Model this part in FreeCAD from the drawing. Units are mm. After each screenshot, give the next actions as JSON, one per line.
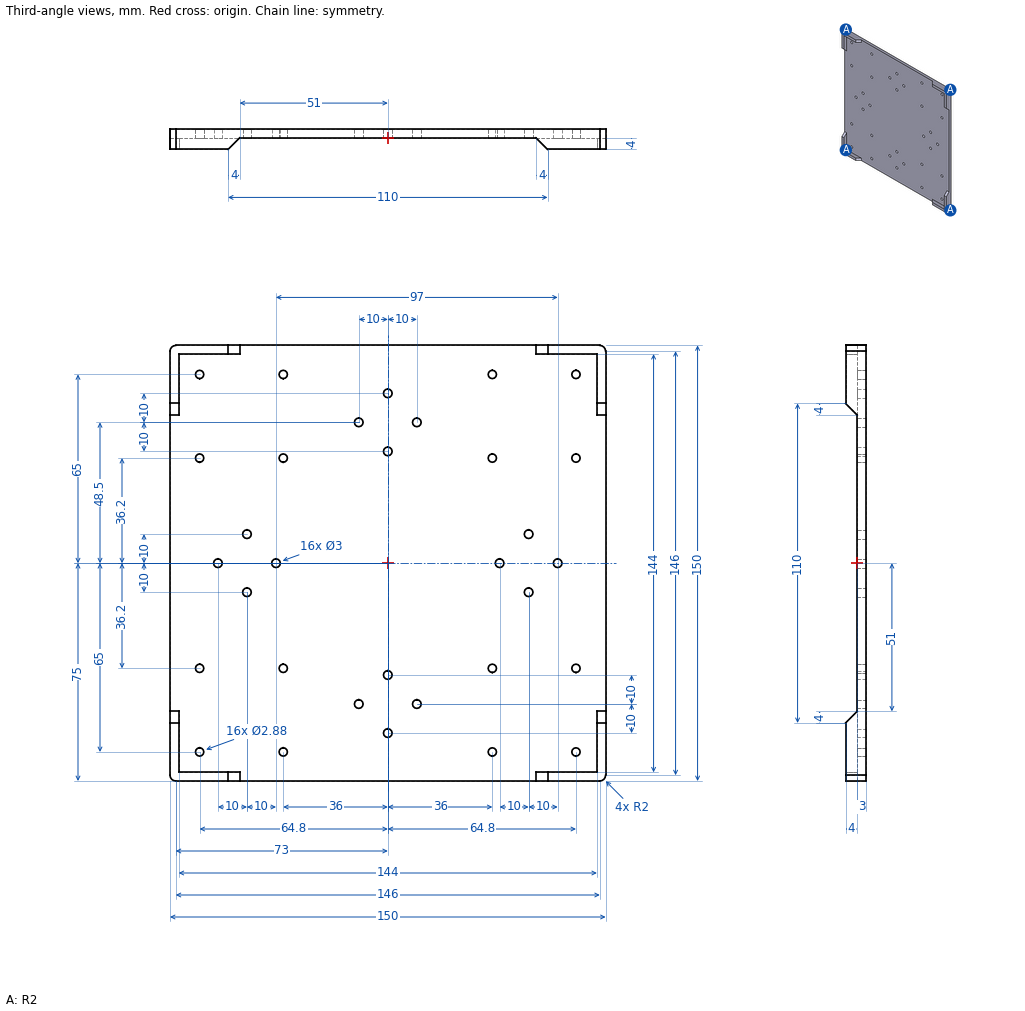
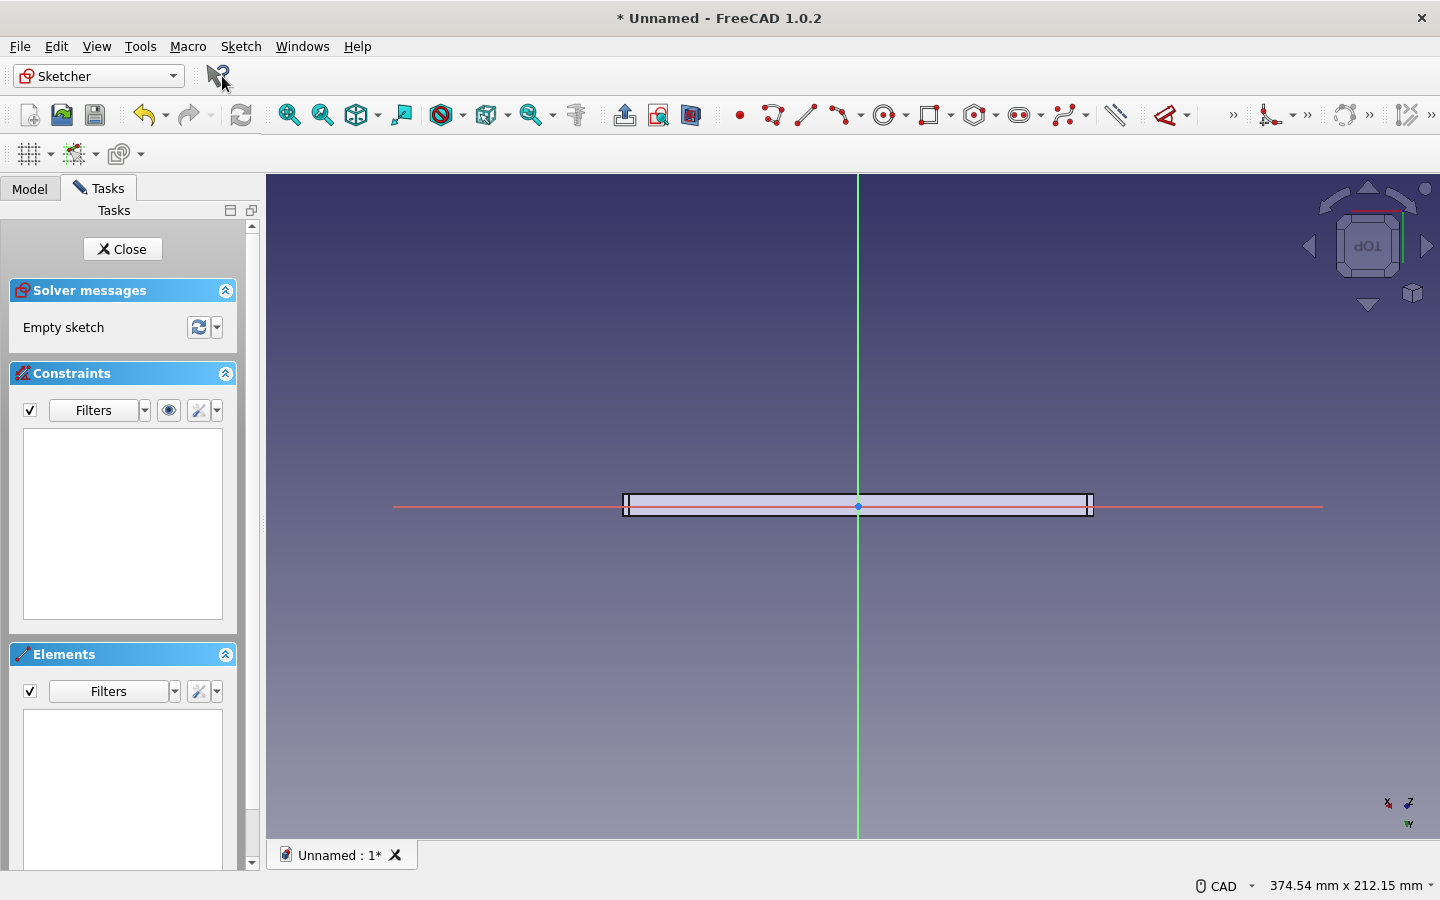
{"action": "scroll", "coordinate": [948, 493], "scroll_direction": "up", "scroll_amount": 3}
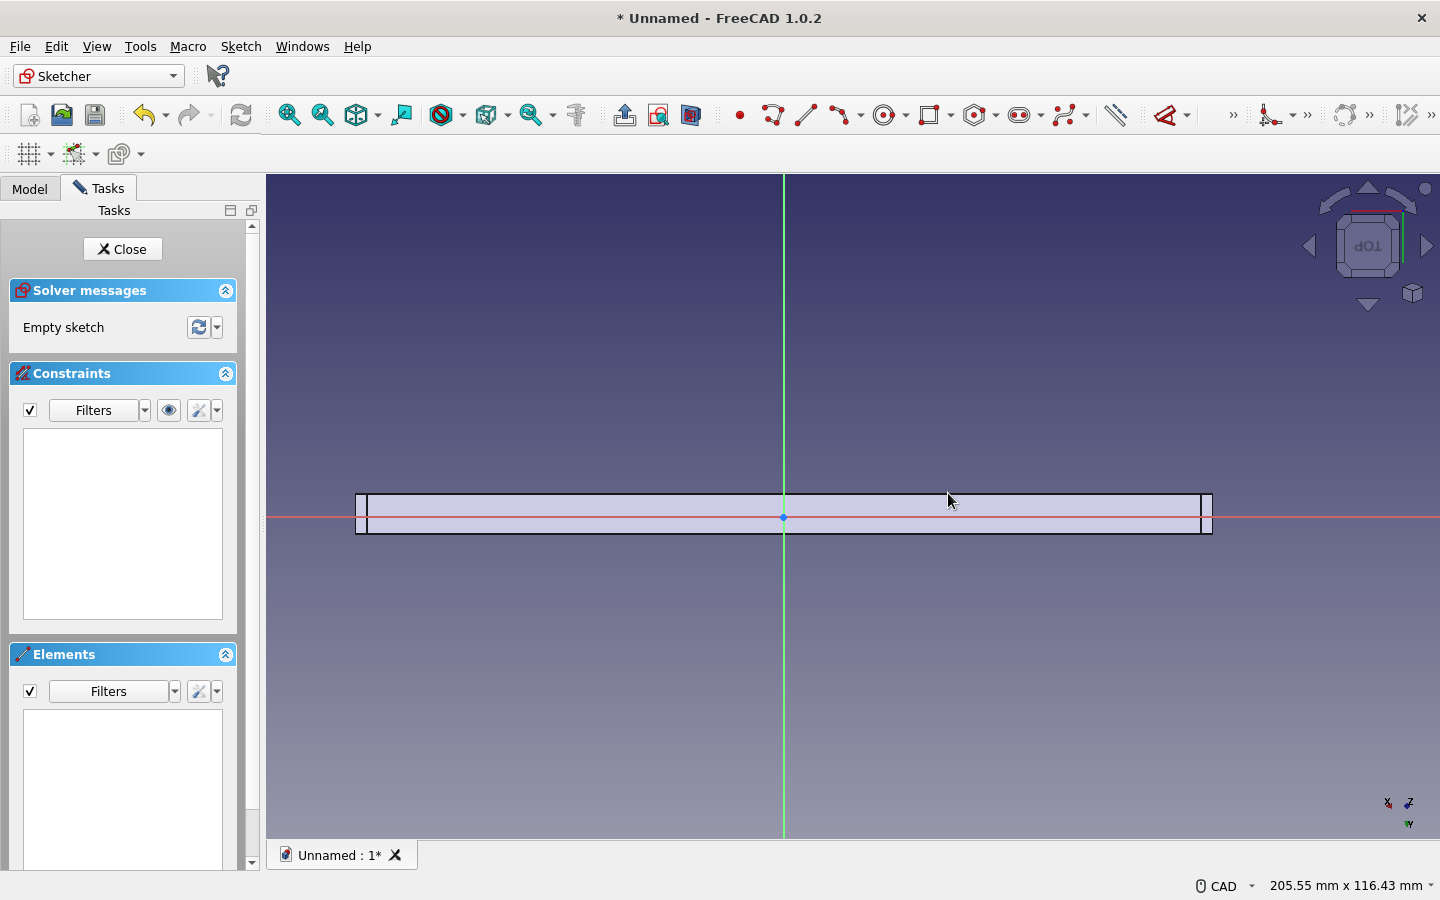
{"action": "key", "text": "g m"}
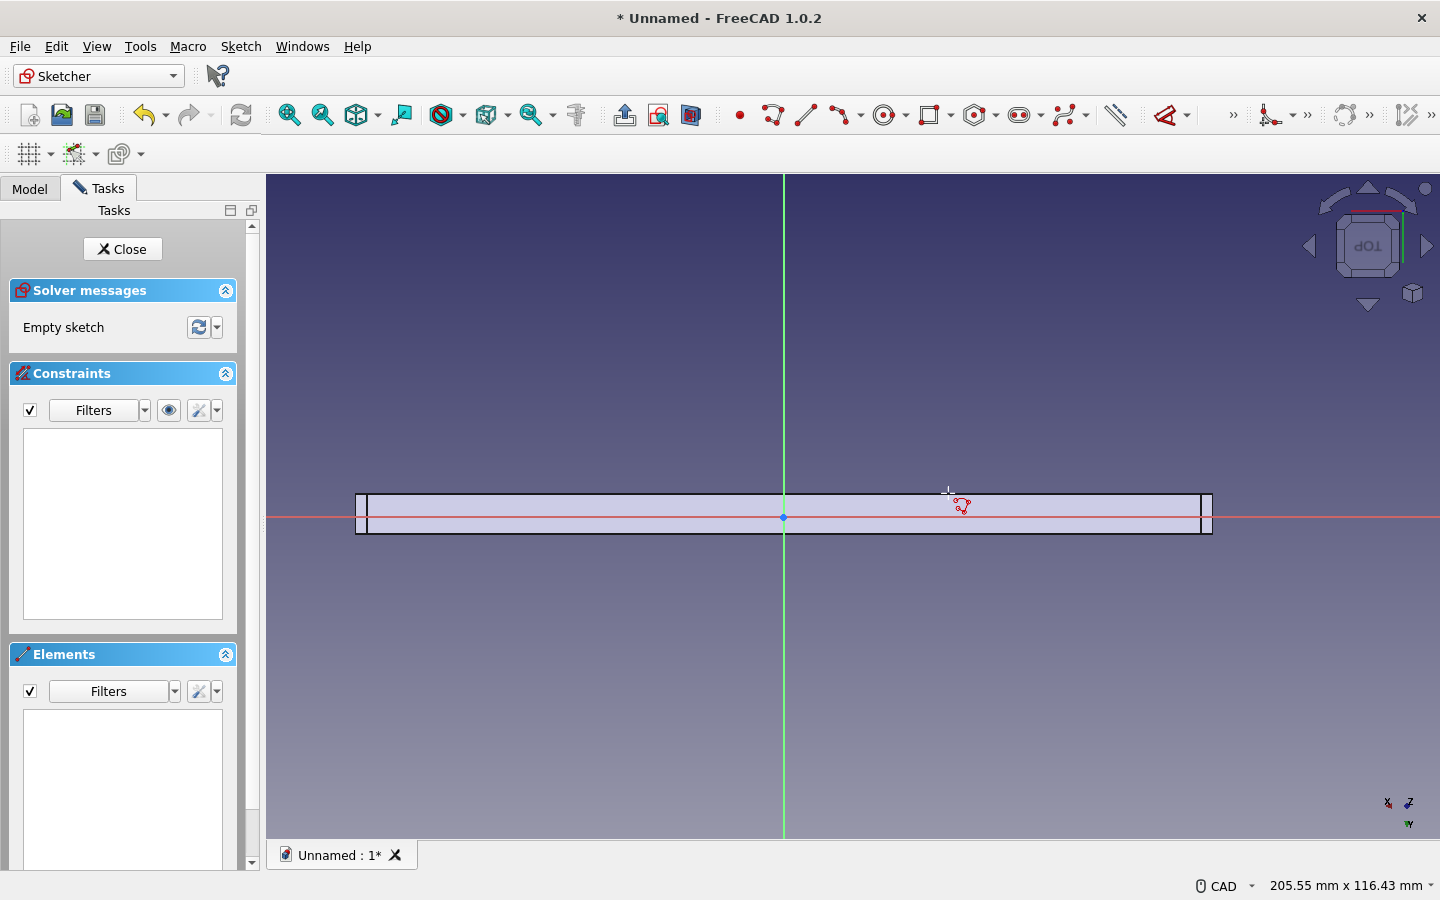
{"action": "left_click", "coordinate": [1075, 517]}
{"action": "left_click", "coordinate": [1098, 494]}
{"action": "left_click", "coordinate": [470, 494]}
{"action": "left_click", "coordinate": [493, 508]}
{"action": "left_click", "coordinate": [1075, 517]}
{"action": "key", "text": "Escape"}
{"action": "key", "text": "Escape"}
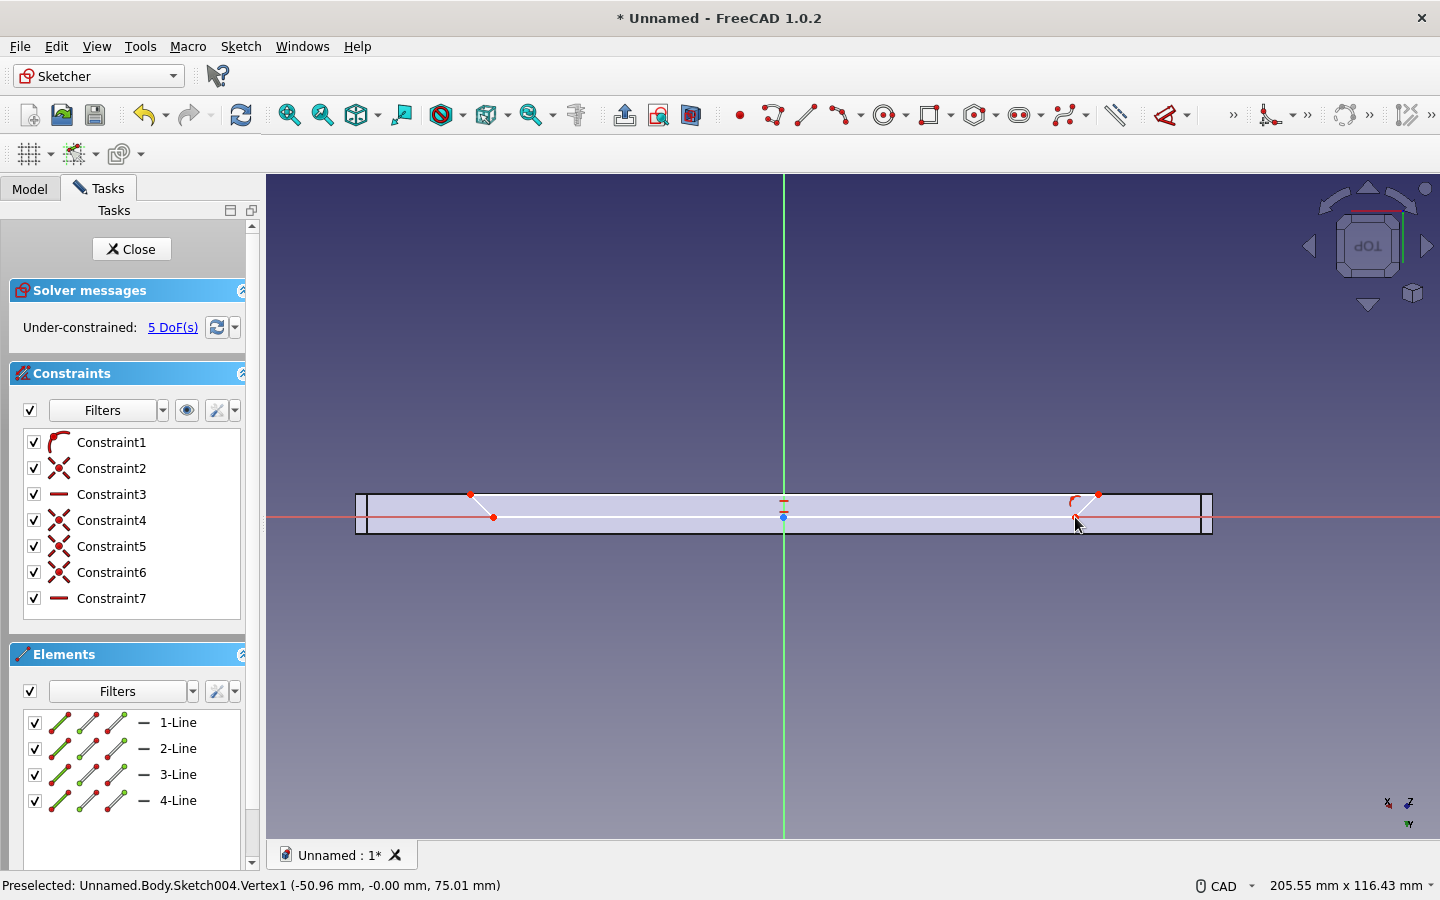
{"action": "left_click", "coordinate": [1164, 116]}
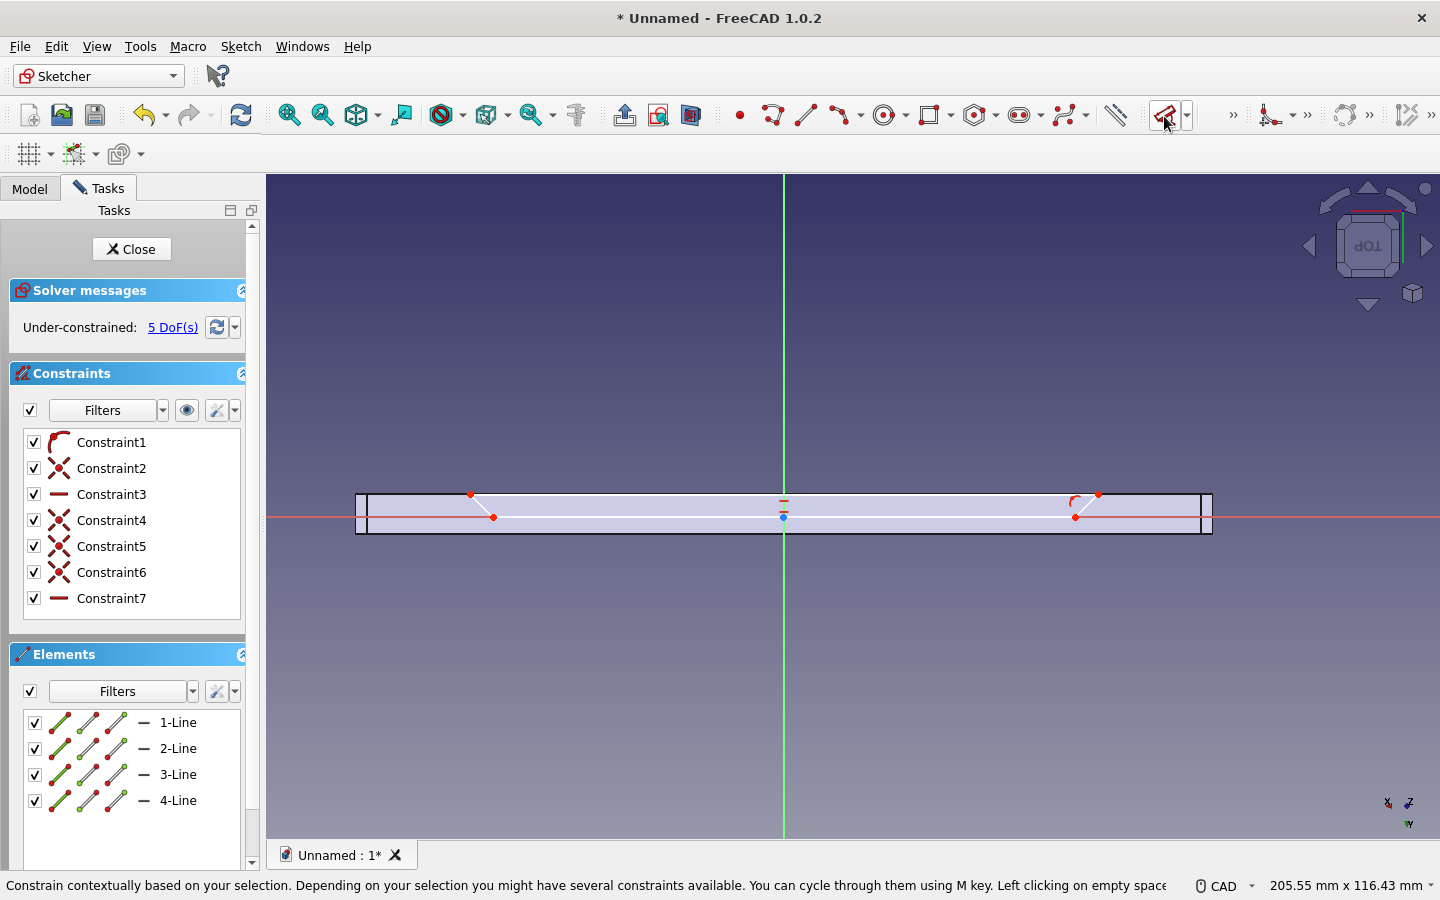
{"action": "scroll", "coordinate": [1098, 495], "scroll_direction": "up", "scroll_amount": 3}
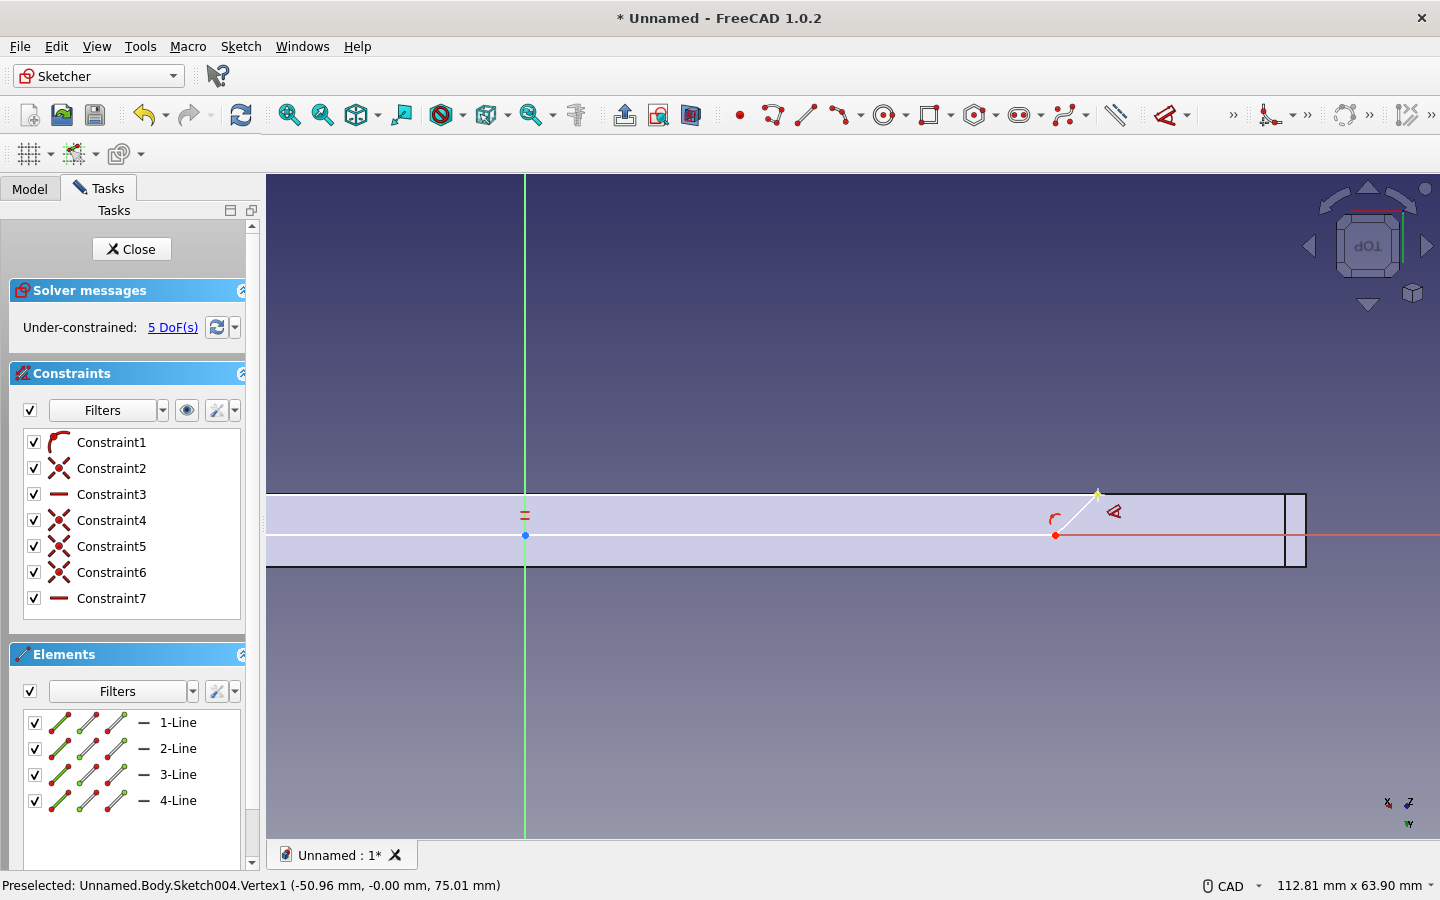
{"action": "left_click", "coordinate": [1097, 495]}
{"action": "left_click", "coordinate": [1131, 515]}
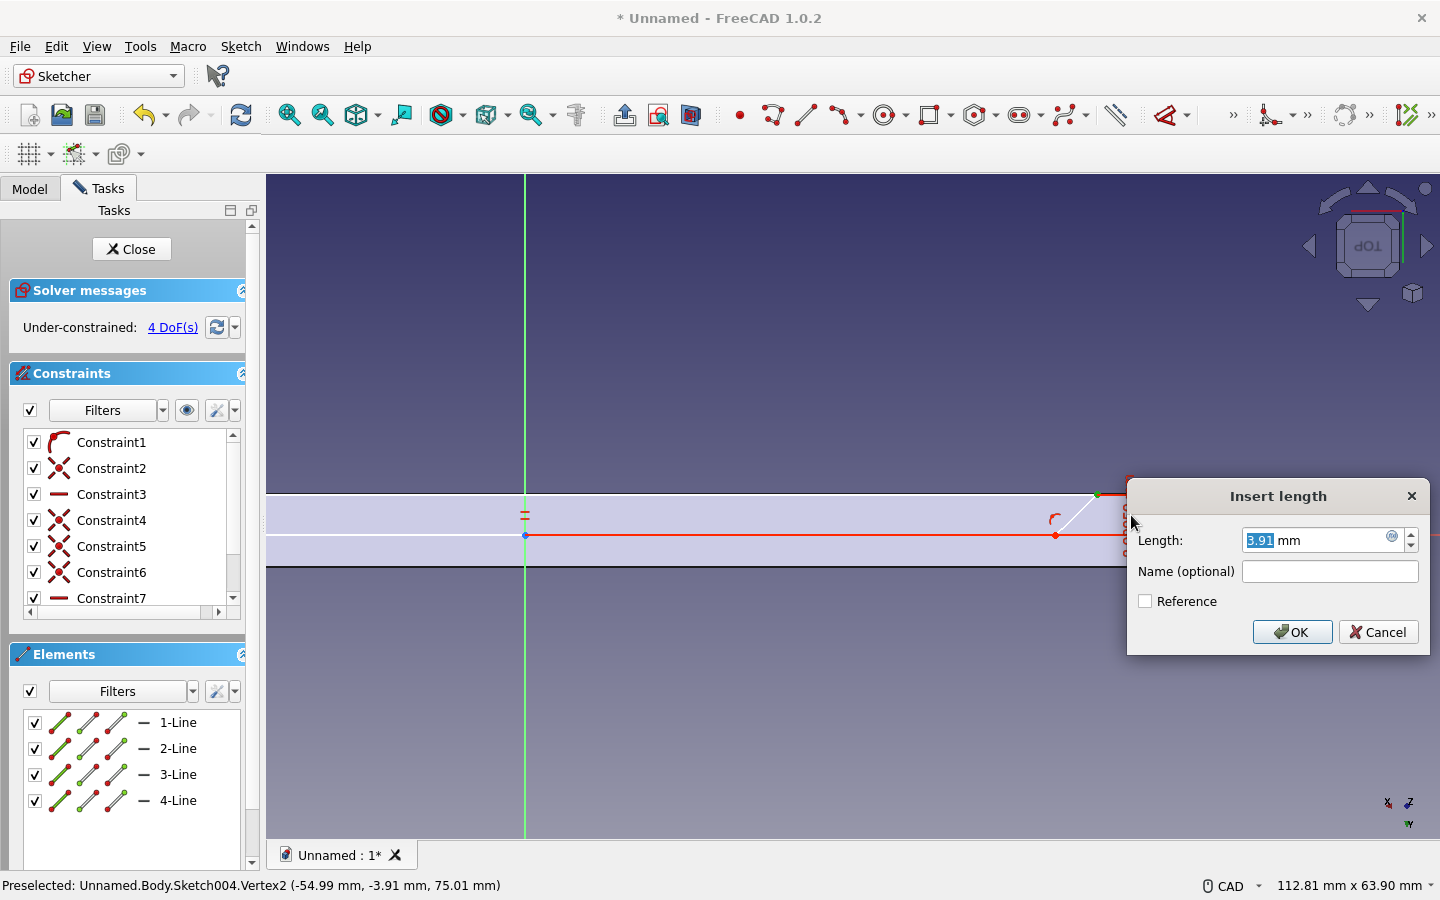
{"action": "type", "text": "4"}
{"action": "key", "text": "Return"}